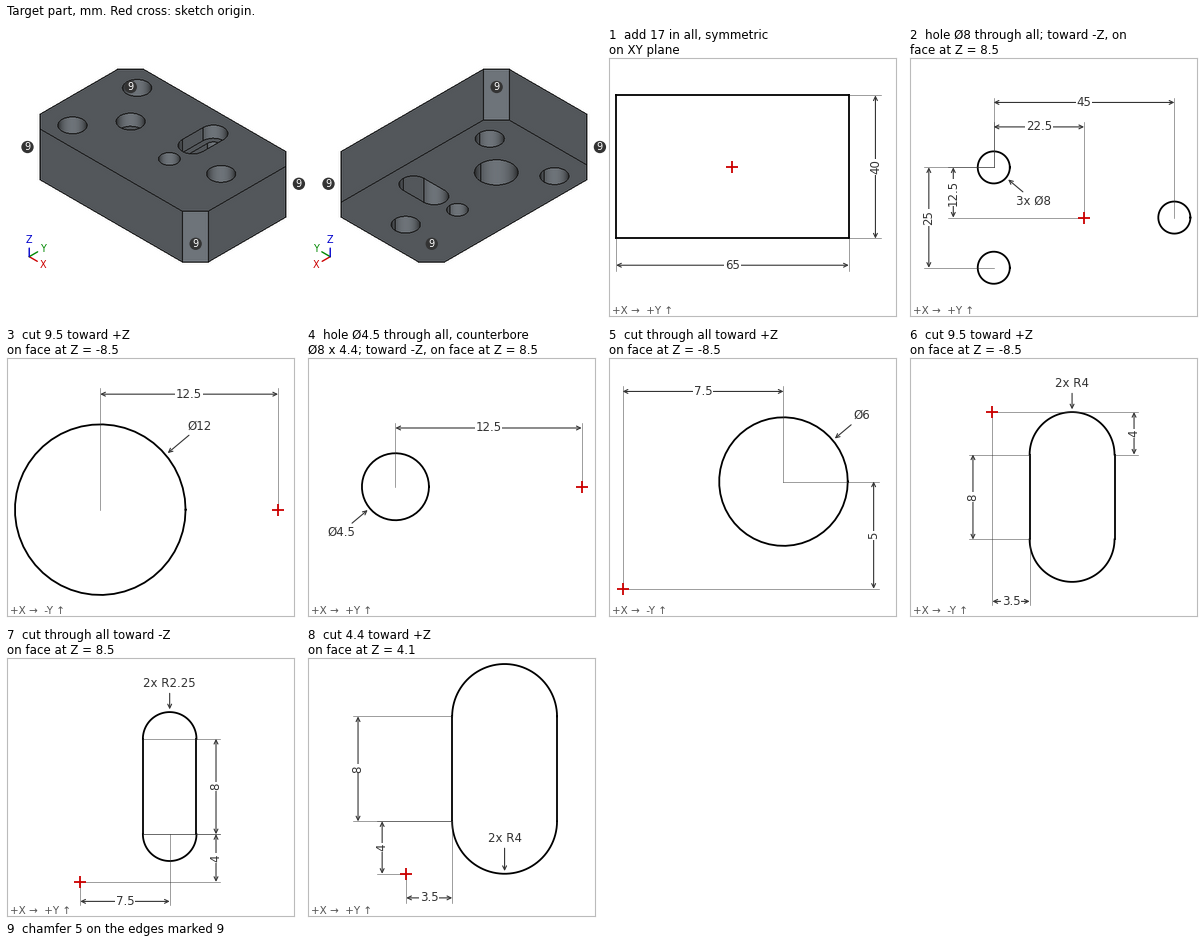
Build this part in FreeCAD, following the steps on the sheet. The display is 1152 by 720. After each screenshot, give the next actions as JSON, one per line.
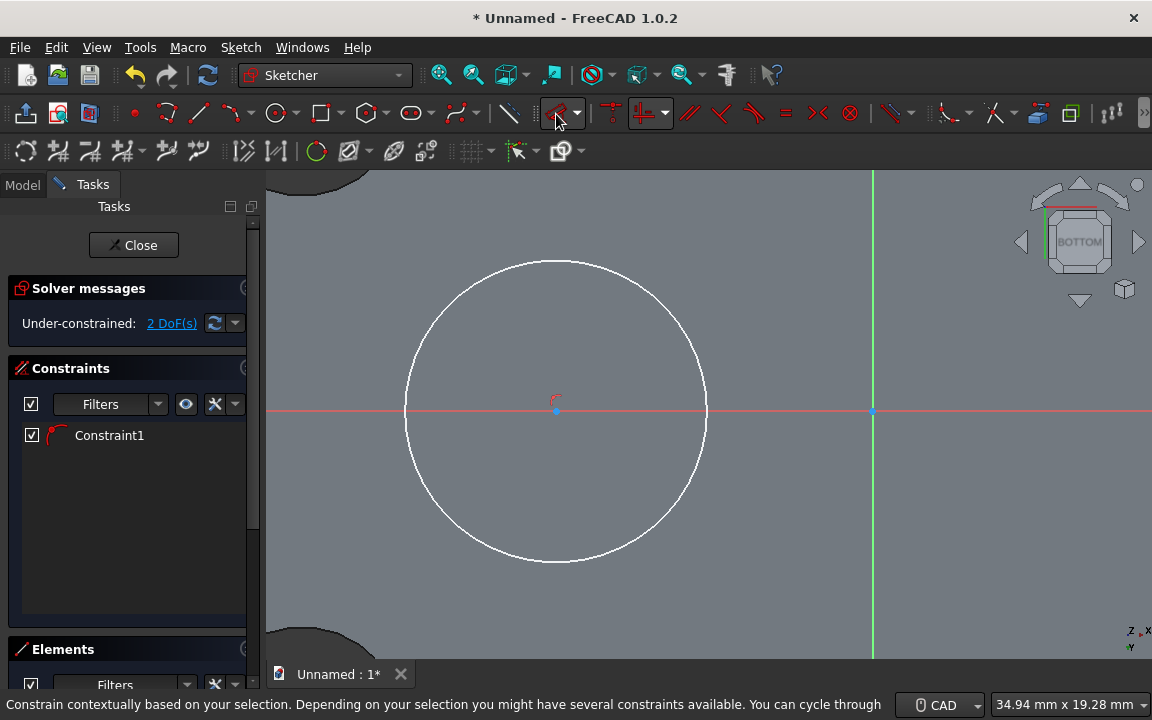
{"action": "left_click", "coordinate": [662, 304]}
{"action": "left_click", "coordinate": [684, 281]}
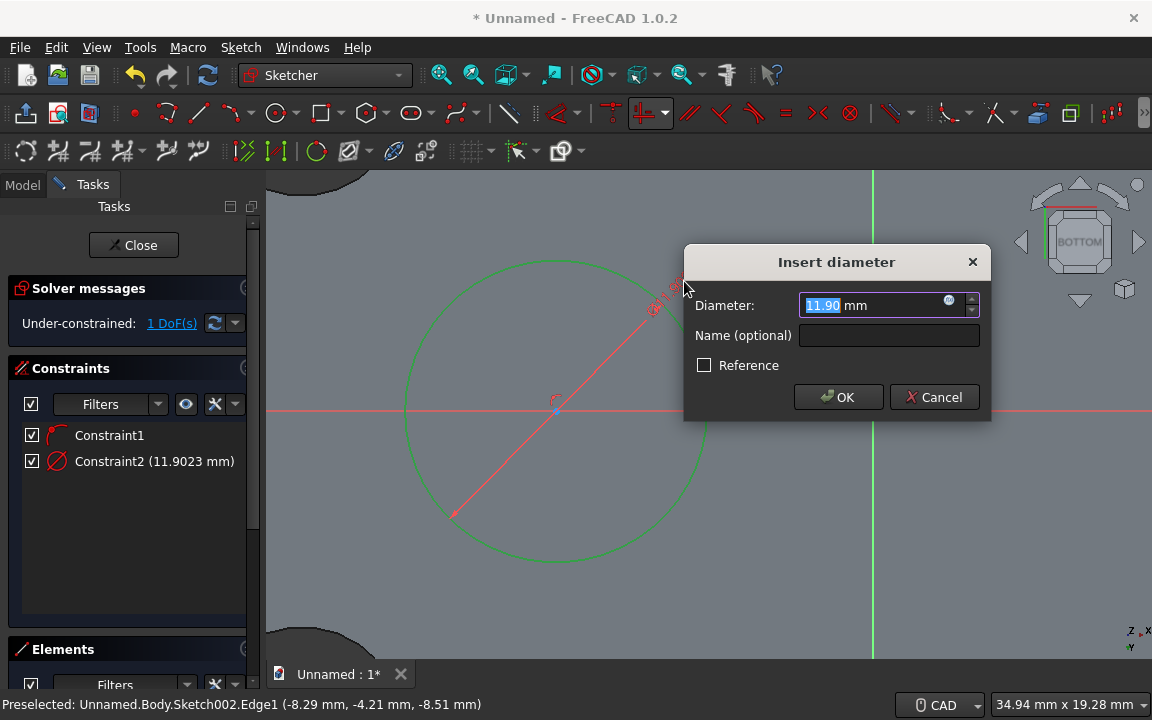
{"action": "type", "text": "12"}
{"action": "key", "text": "Return"}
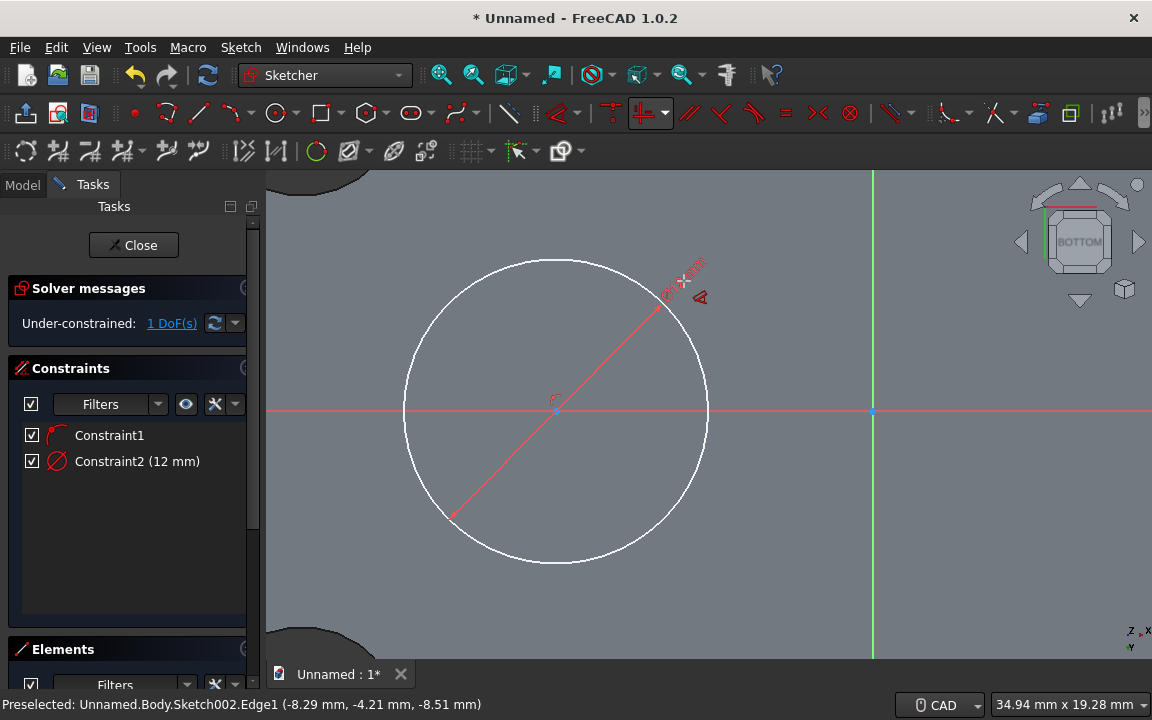
{"action": "left_click", "coordinate": [556, 411]}
{"action": "left_click", "coordinate": [641, 445]}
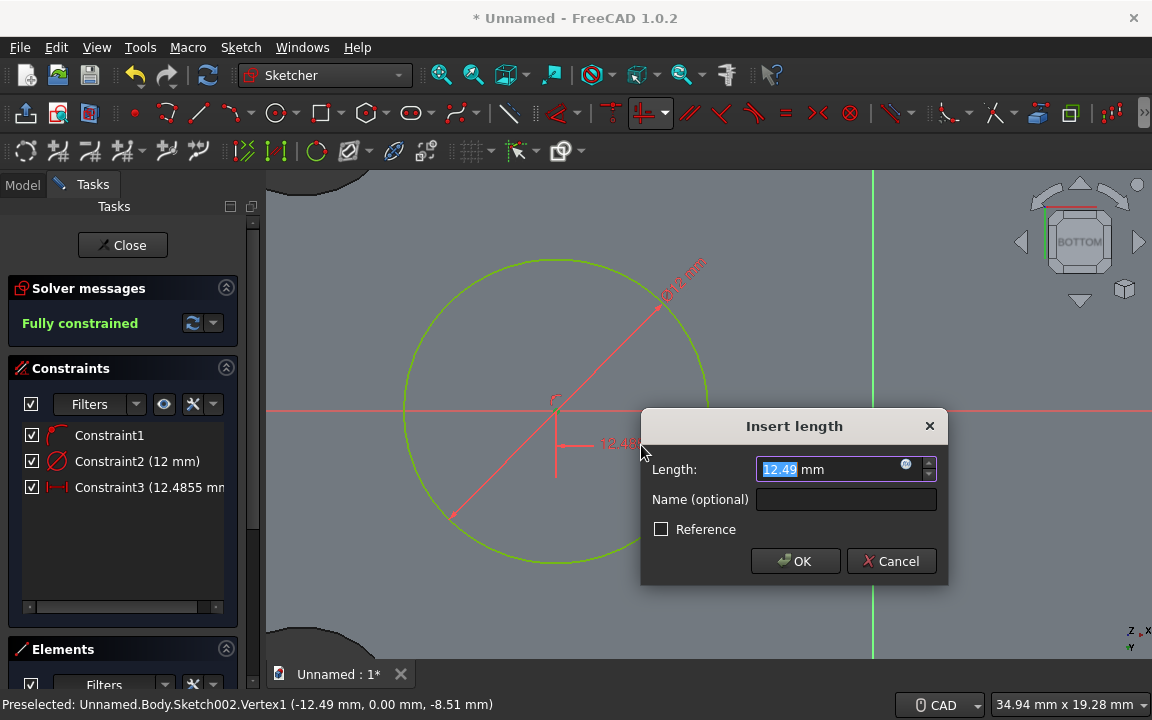
{"action": "type", "text": "12.5"}
{"action": "key", "text": "Return"}
{"action": "key", "text": "Escape"}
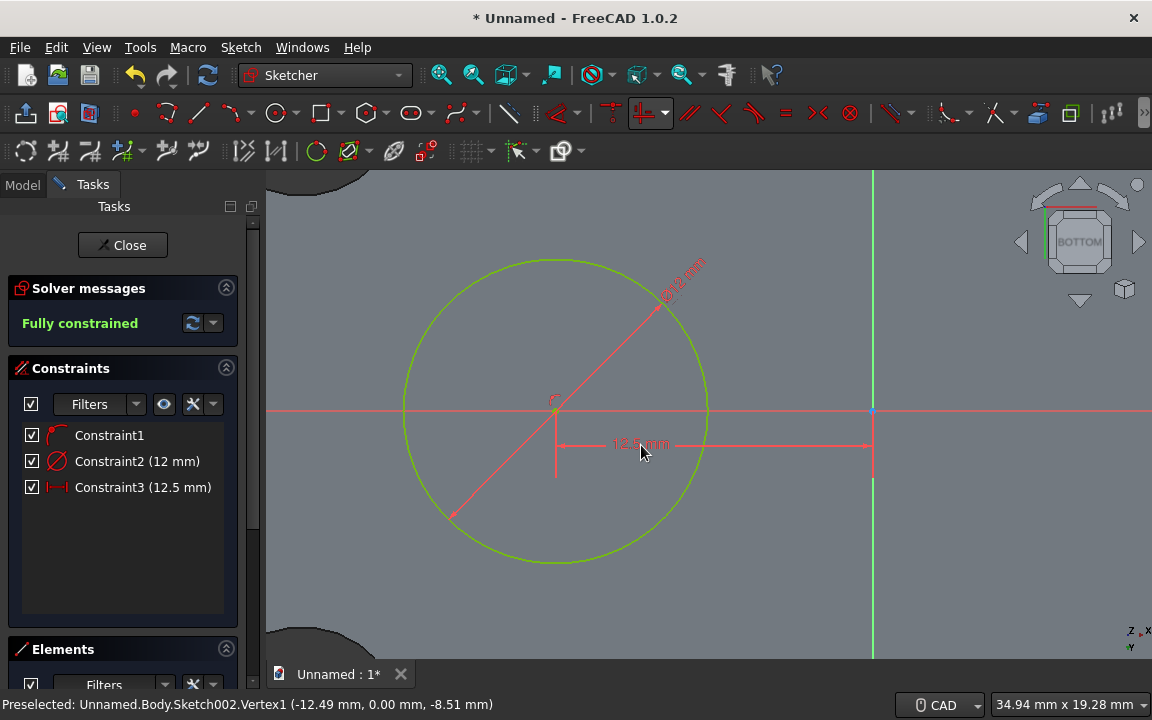
{"action": "left_click", "coordinate": [123, 245]}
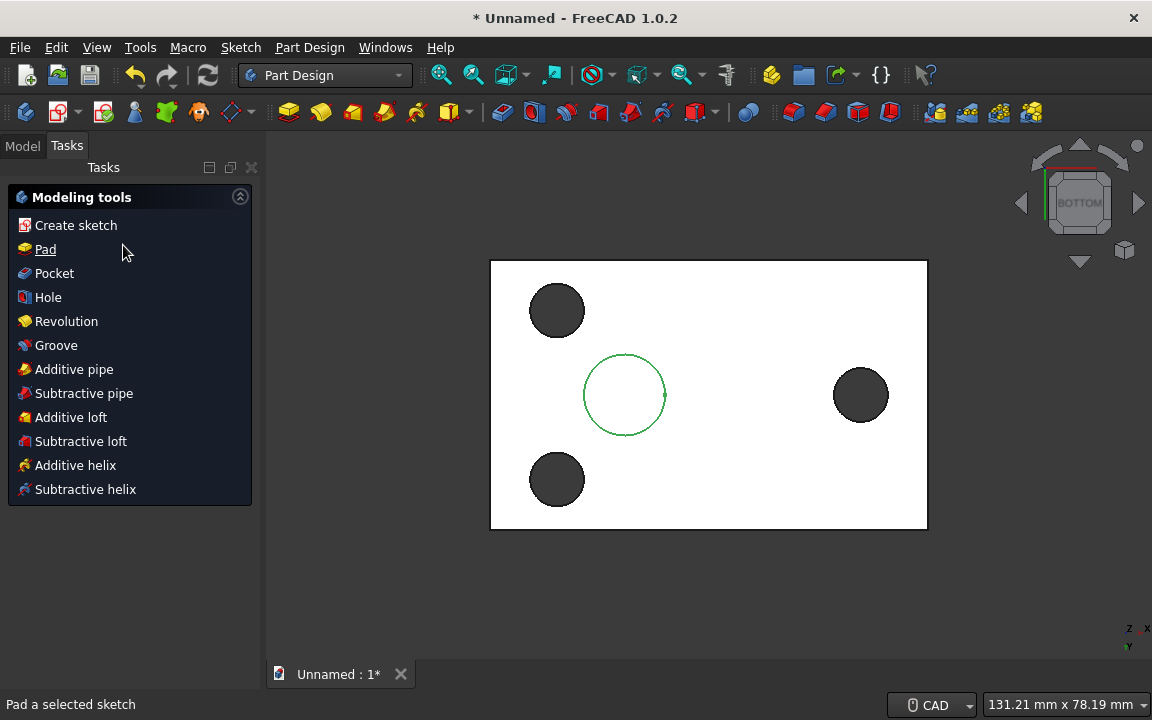
{"action": "left_click", "coordinate": [504, 112]}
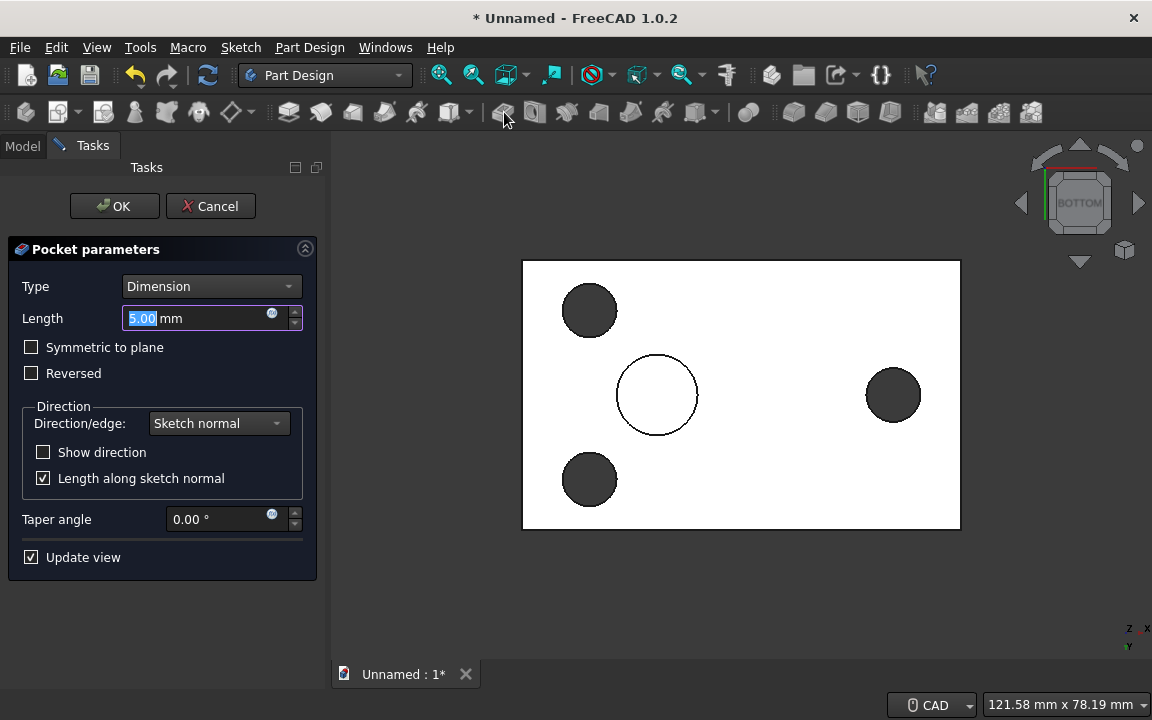
{"action": "type", "text": "9.5"}
{"action": "key", "text": "Tab"}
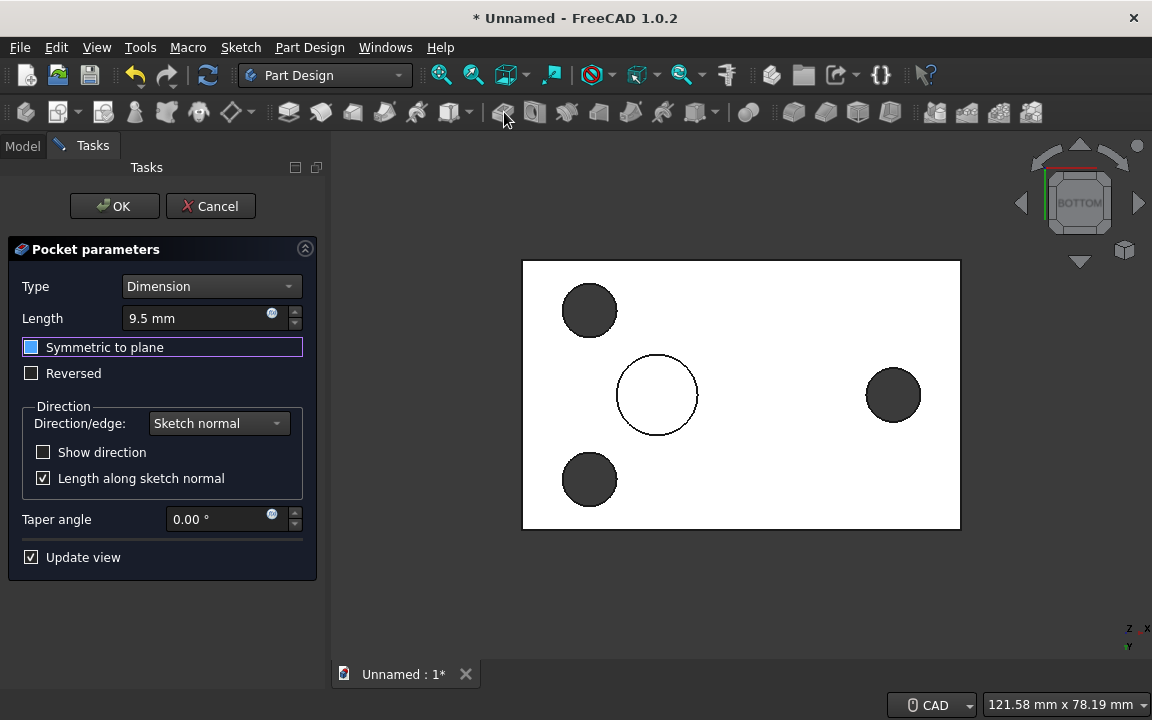
{"action": "left_click", "coordinate": [115, 206]}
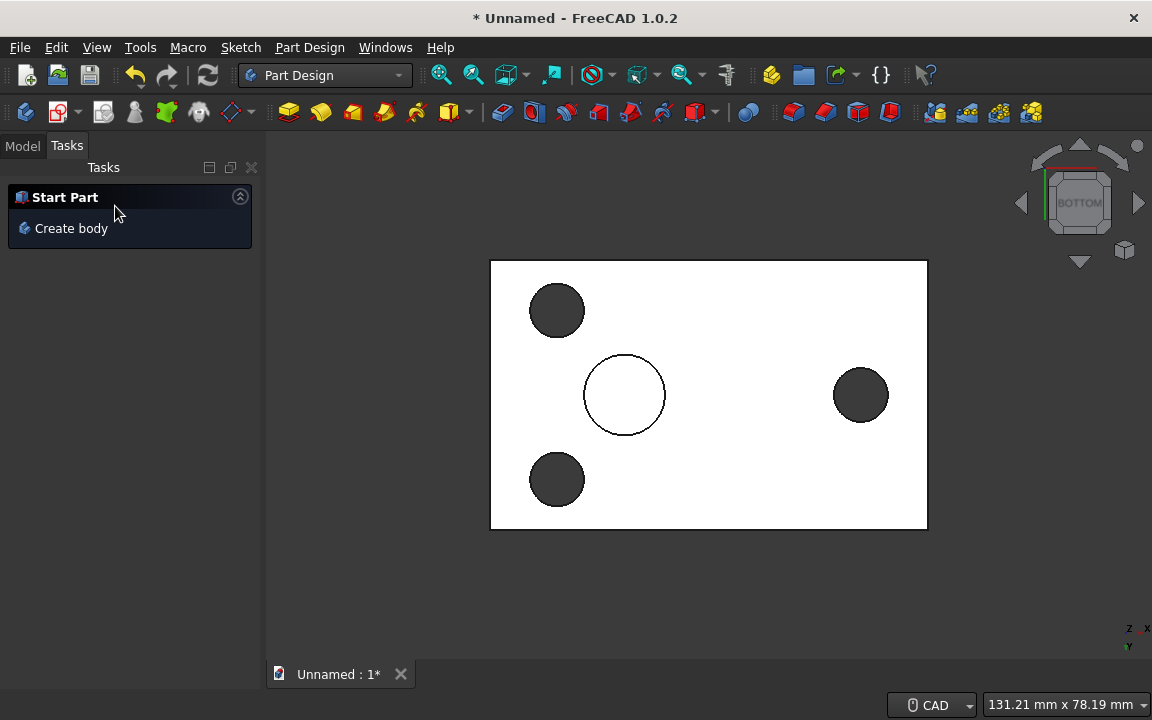
{"action": "key", "text": "0"}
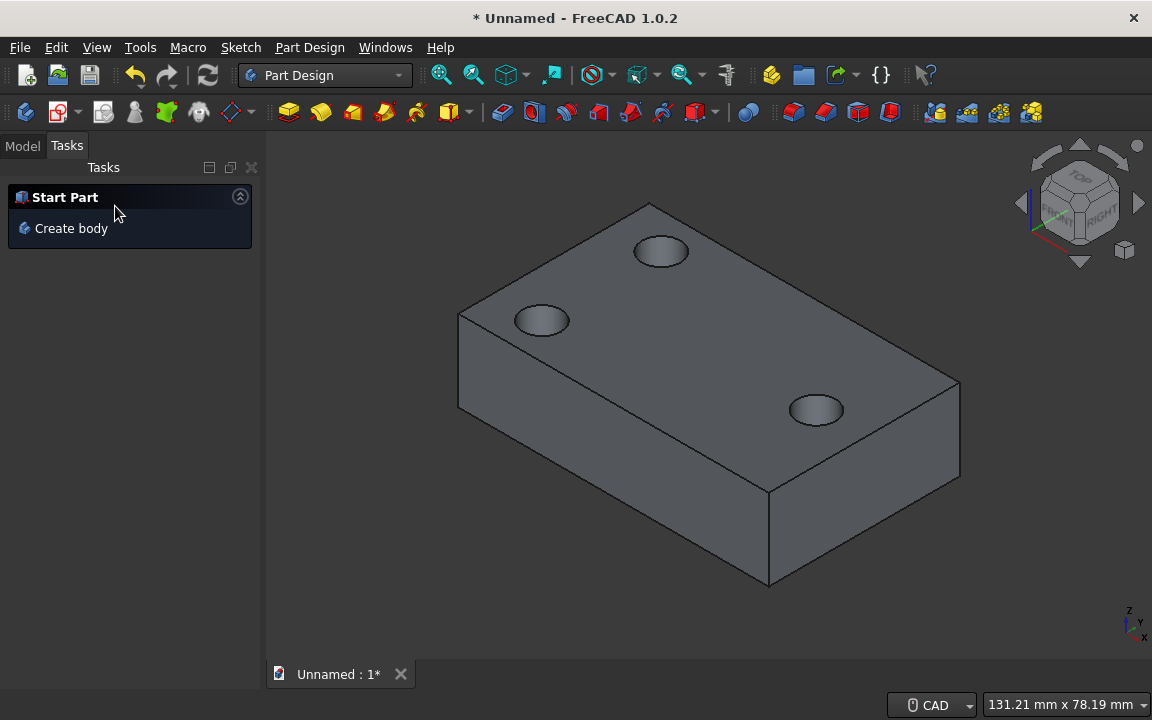
{"action": "left_click", "coordinate": [709, 347]}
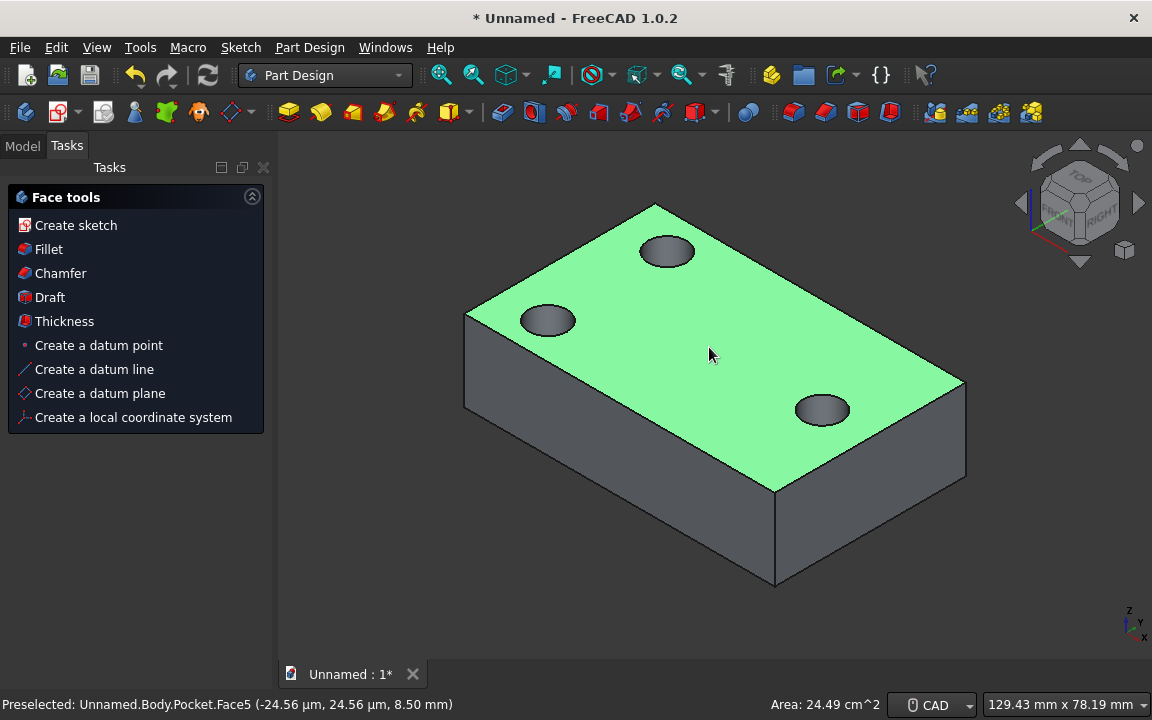
{"action": "left_click", "coordinate": [58, 112]}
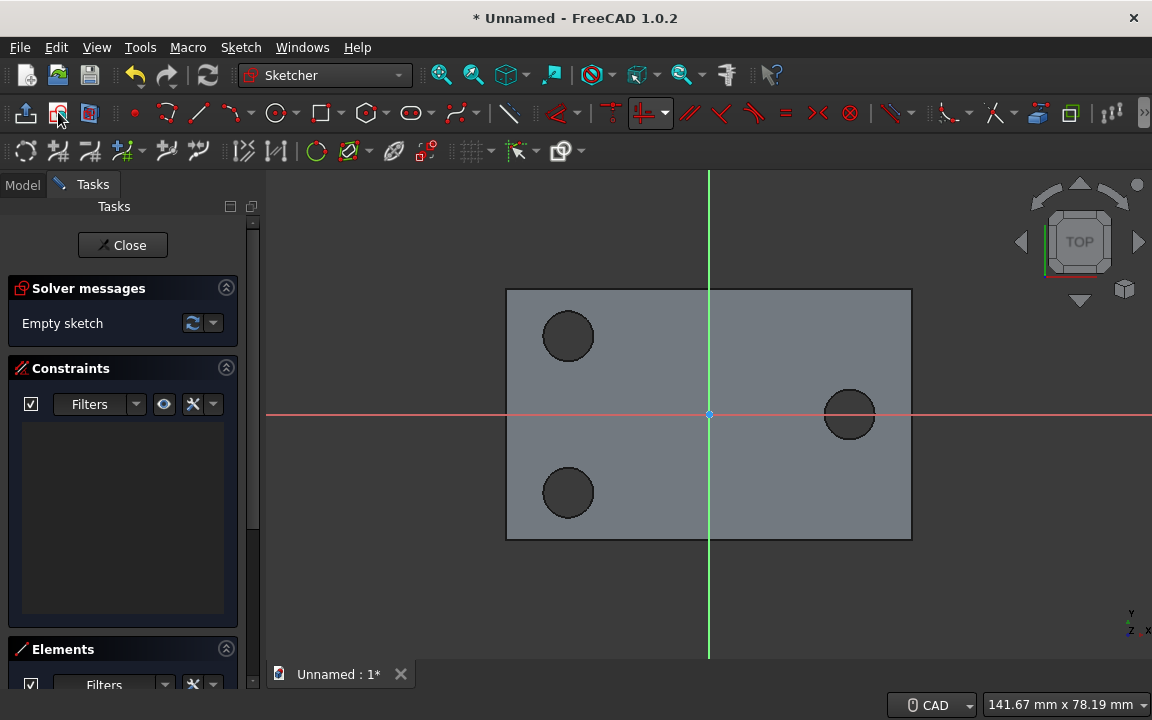
{"action": "scroll", "coordinate": [630, 414], "scroll_direction": "up", "scroll_amount": 12}